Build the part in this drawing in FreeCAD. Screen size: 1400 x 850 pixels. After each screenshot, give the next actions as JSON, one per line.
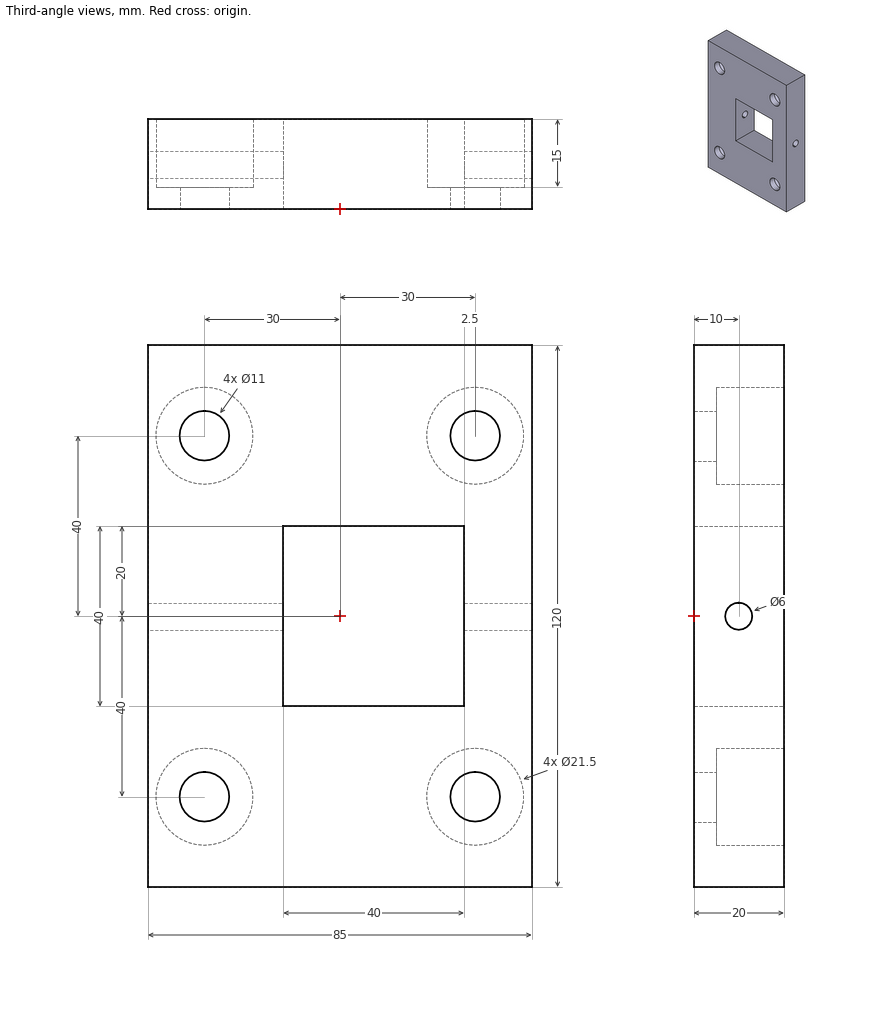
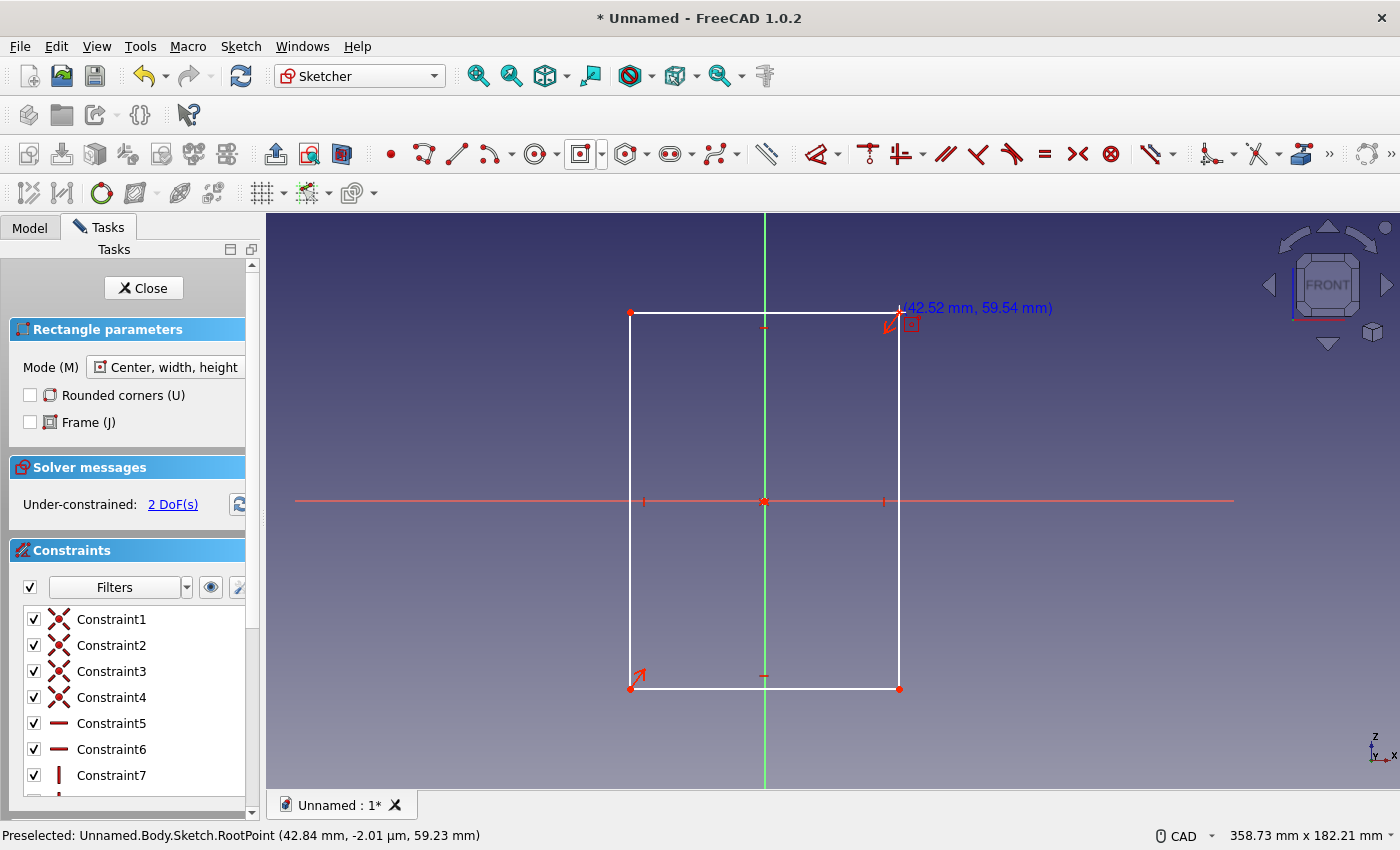
{"action": "key", "text": "g r"}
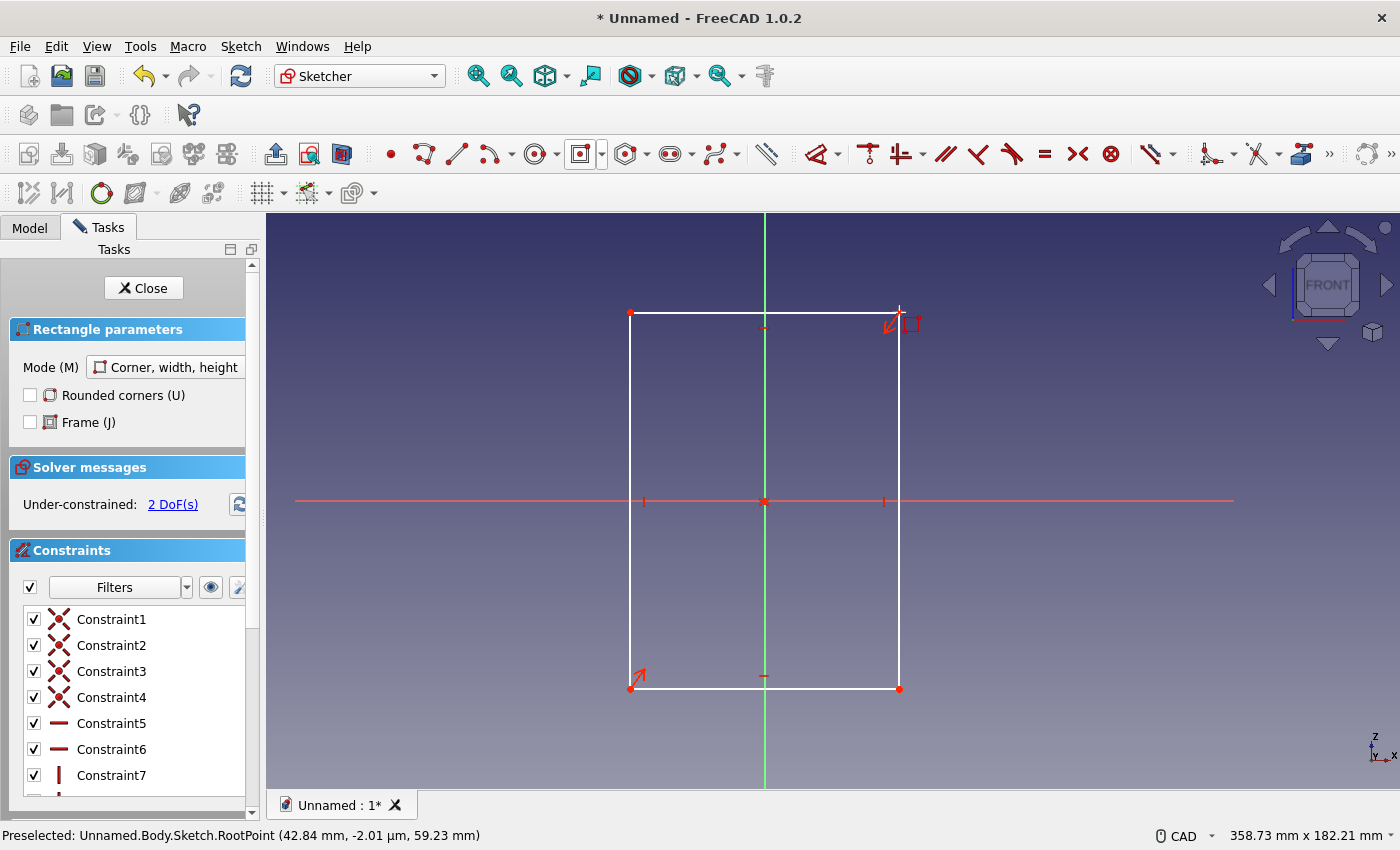
{"action": "left_click", "coordinate": [725, 438]}
{"action": "left_click", "coordinate": [852, 564]}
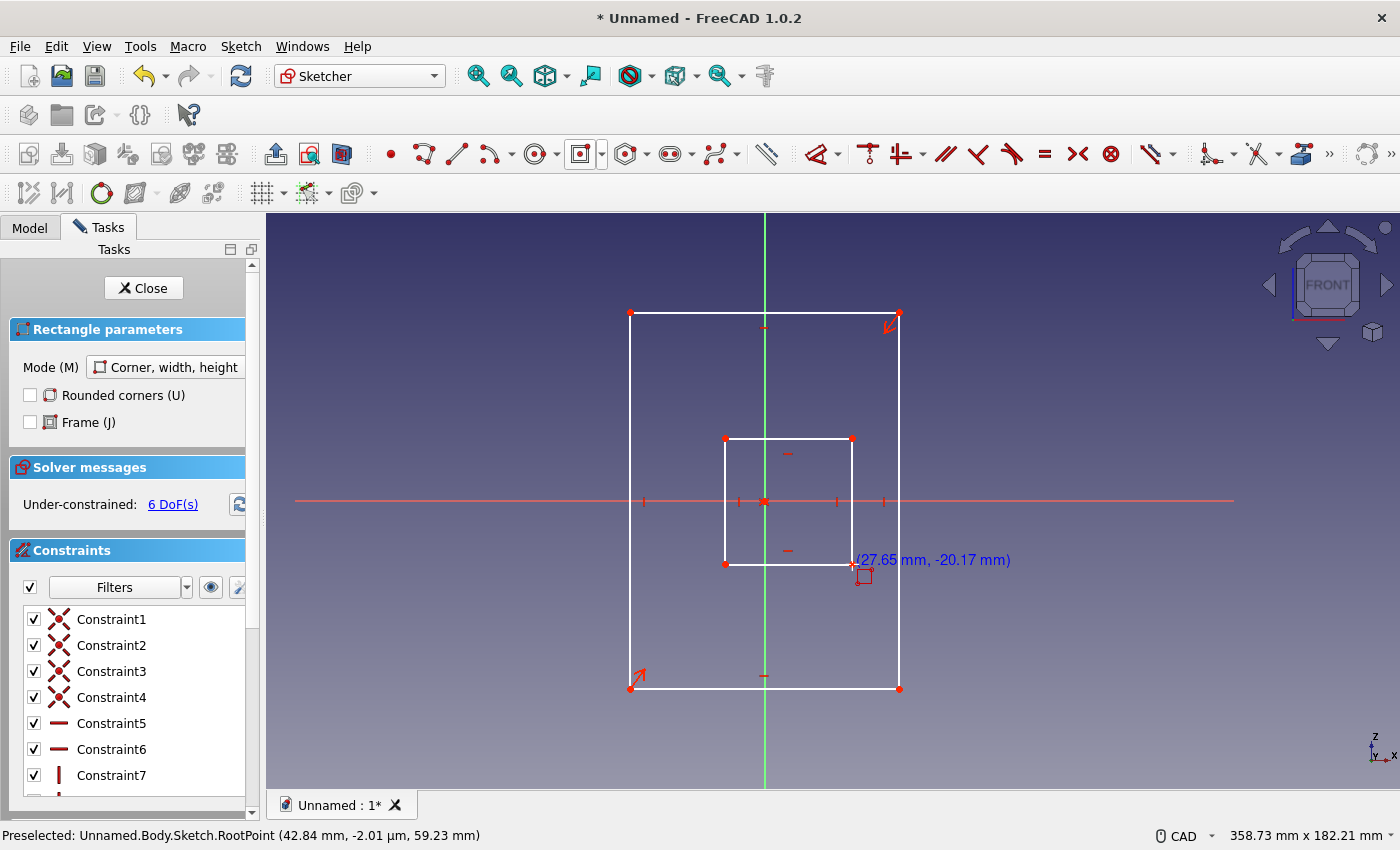
{"action": "key", "text": "g c"}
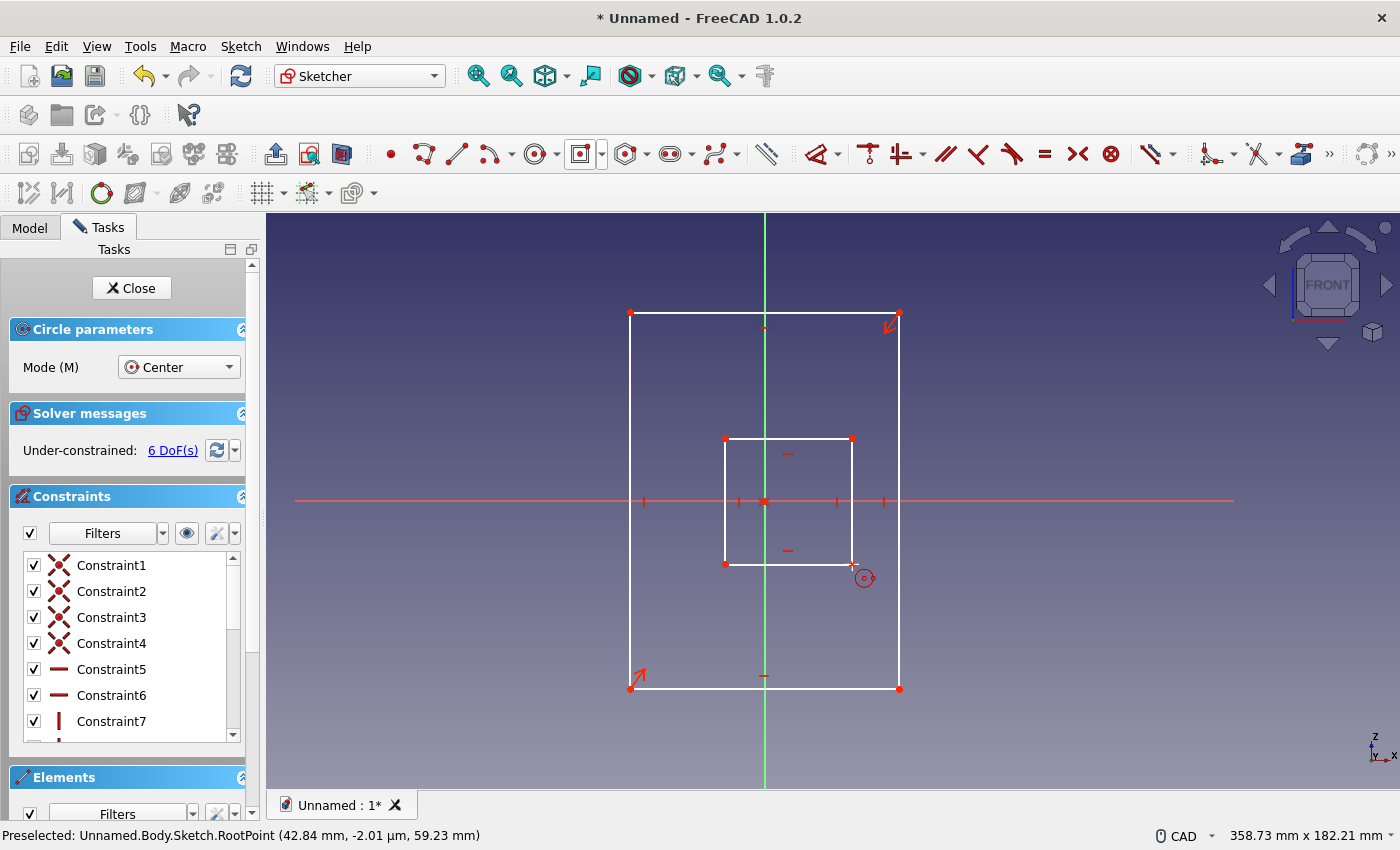
{"action": "scroll", "coordinate": [670, 375], "scroll_direction": "up", "scroll_amount": 2}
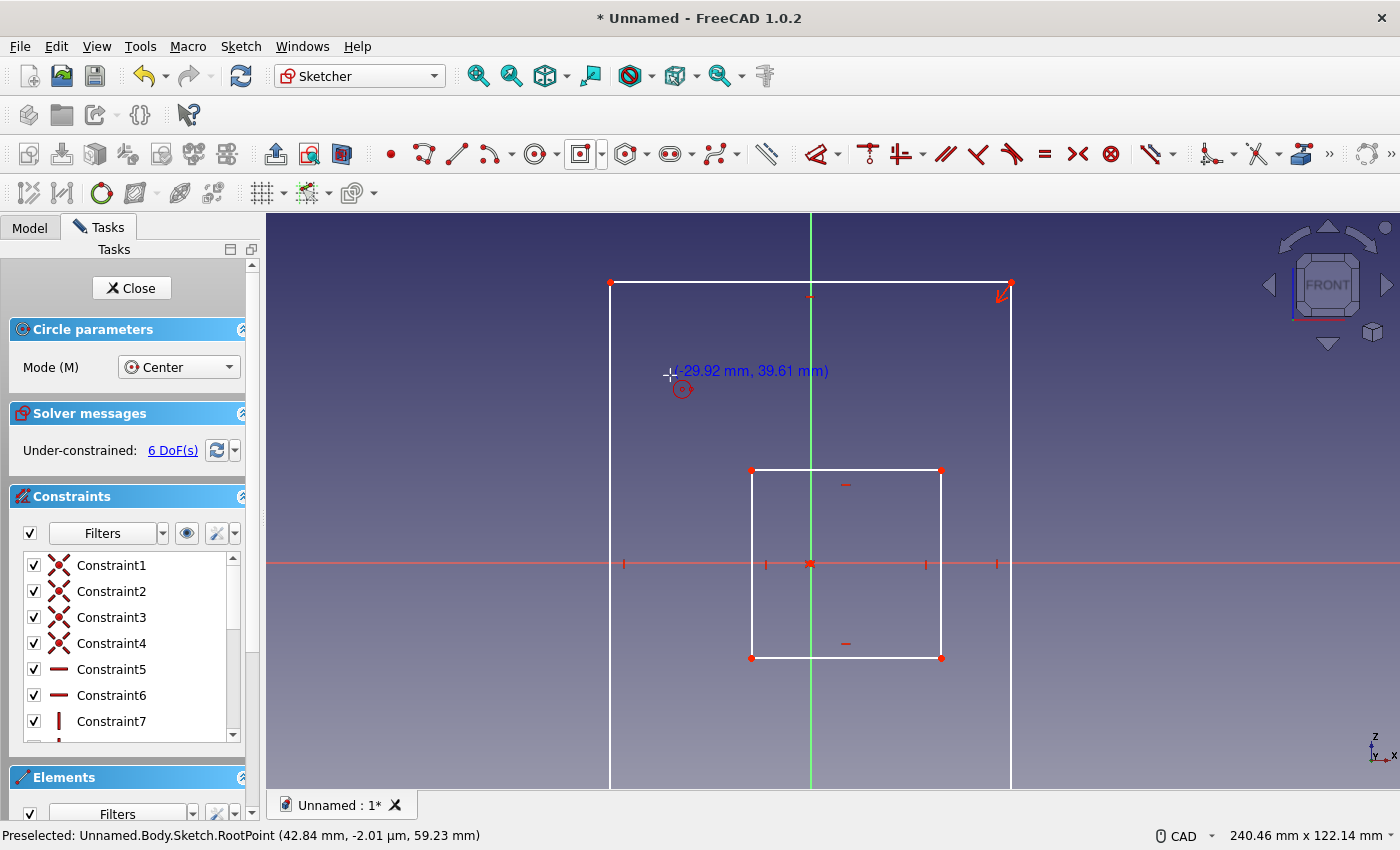
{"action": "left_click", "coordinate": [669, 375]}
{"action": "left_click", "coordinate": [688, 356]}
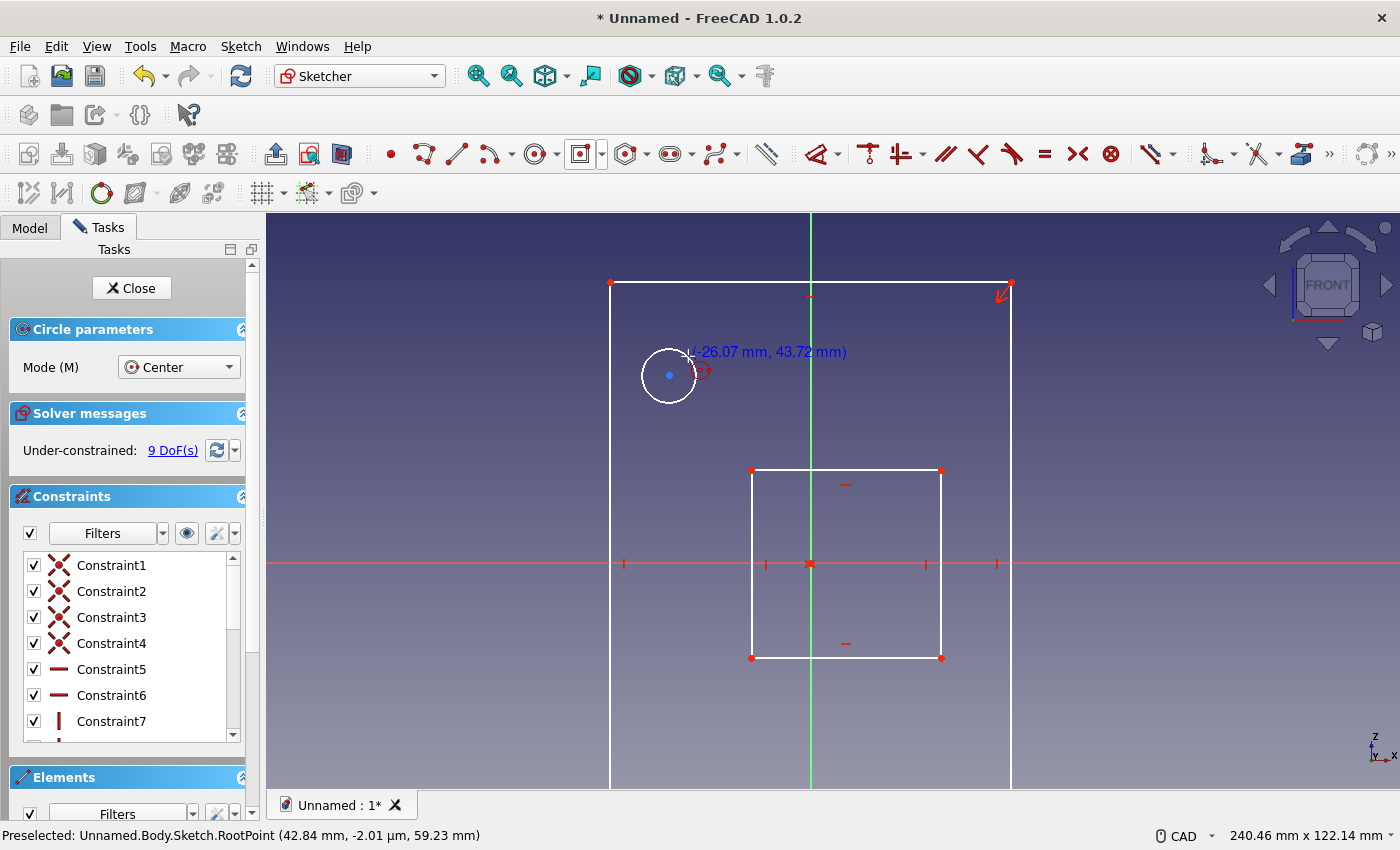
{"action": "left_click", "coordinate": [952, 375]}
{"action": "left_click", "coordinate": [971, 356]}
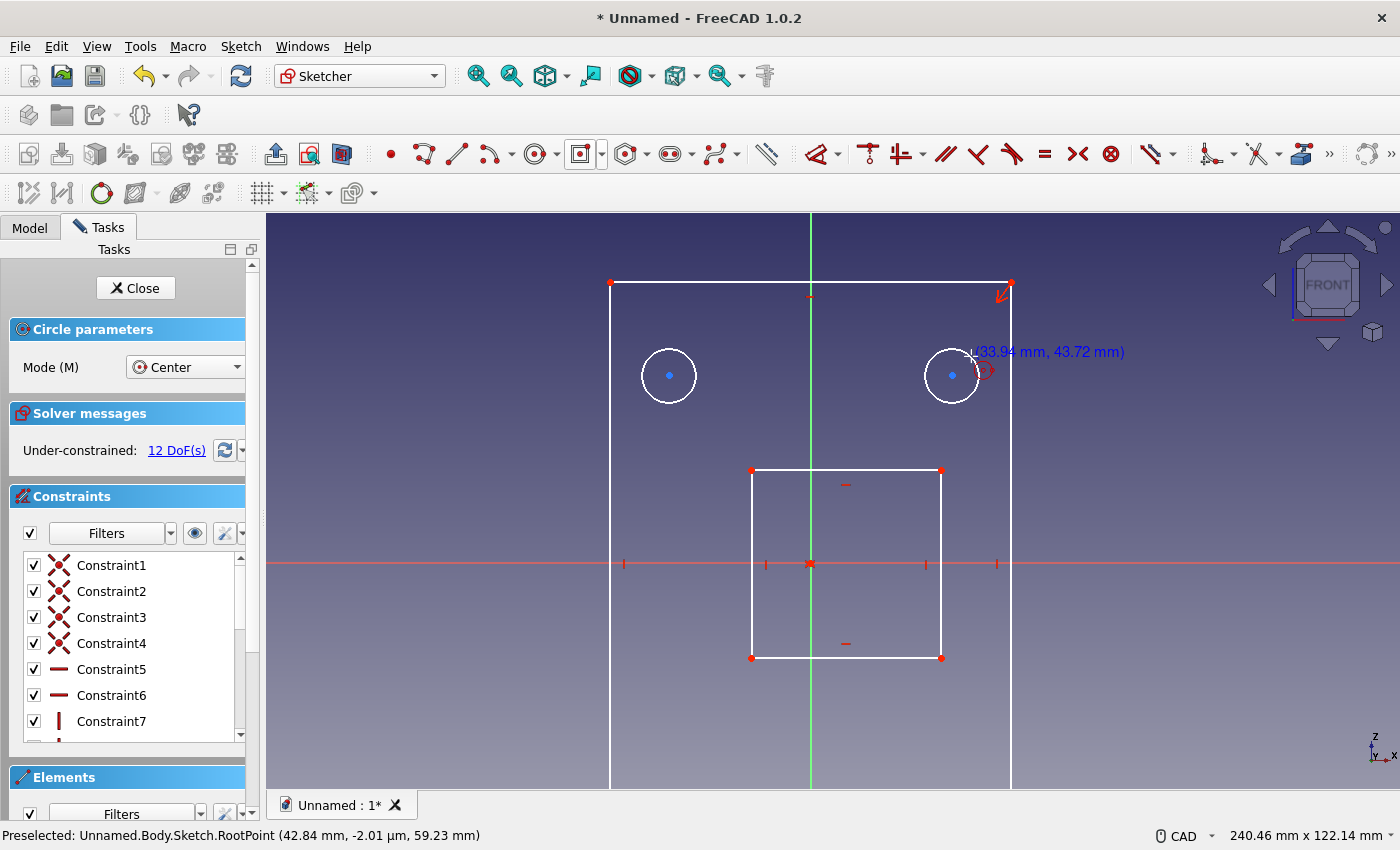
{"action": "left_click", "coordinate": [669, 752]}
{"action": "left_click", "coordinate": [688, 733]}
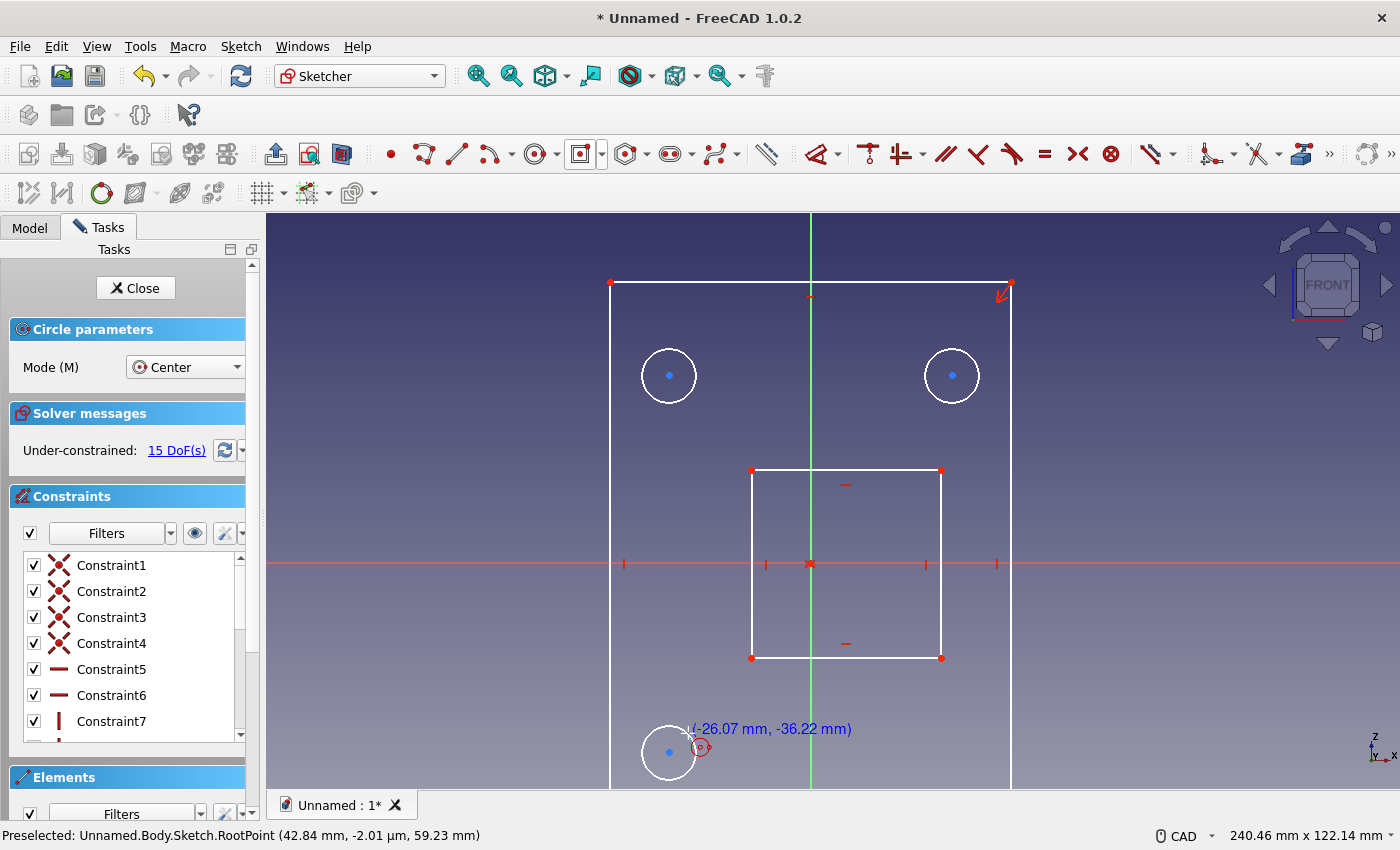
{"action": "left_click", "coordinate": [952, 752]}
{"action": "left_click", "coordinate": [971, 733]}
{"action": "key", "text": "Escape"}